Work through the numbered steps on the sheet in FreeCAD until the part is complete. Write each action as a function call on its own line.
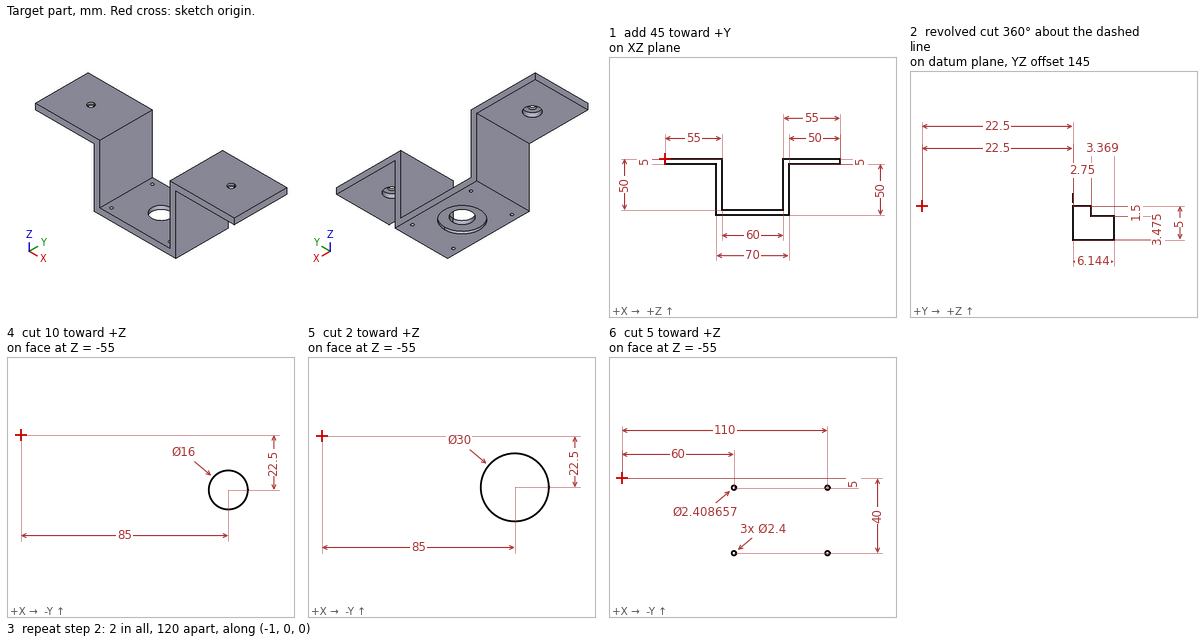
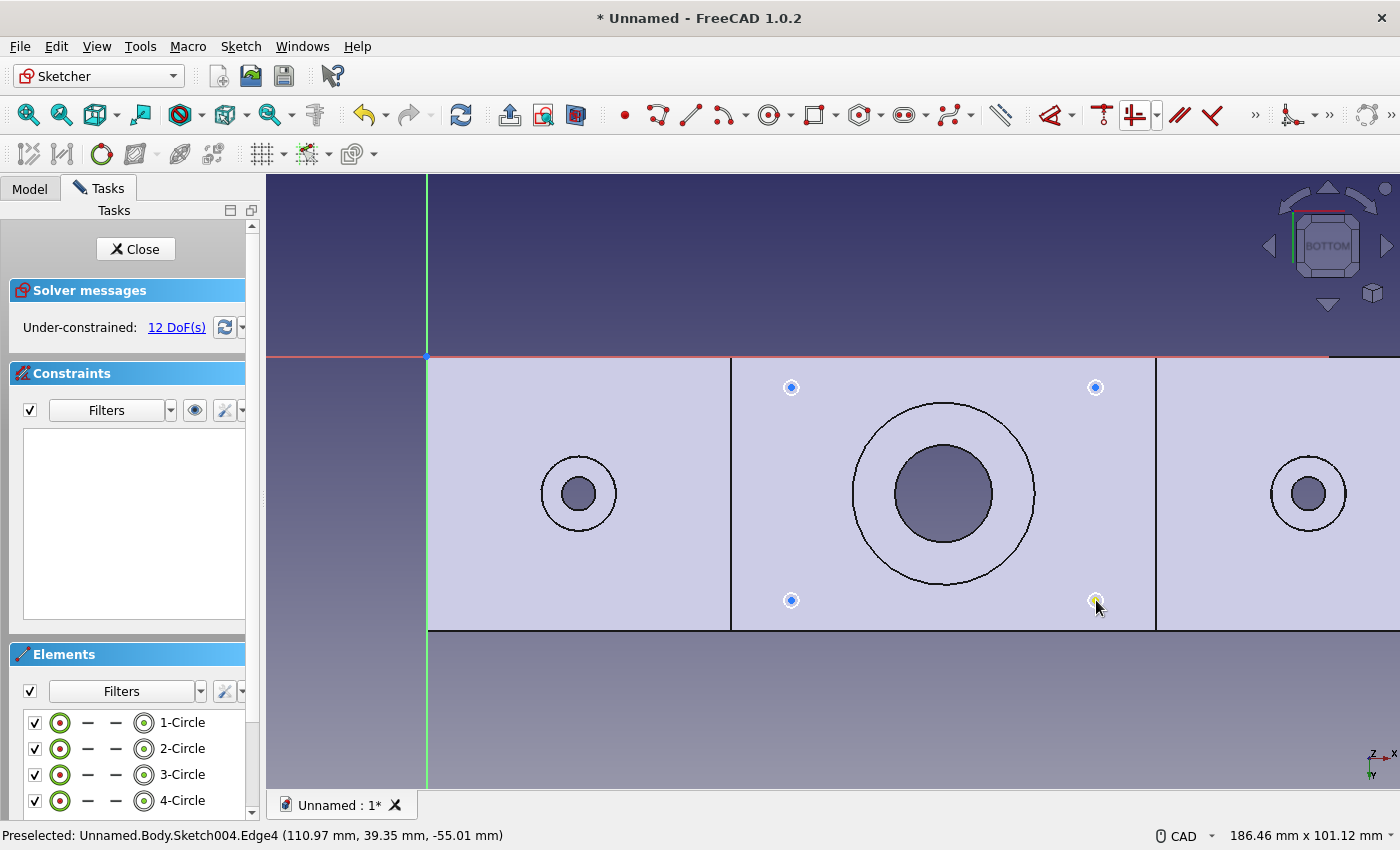
scroll(797, 595, up, 4)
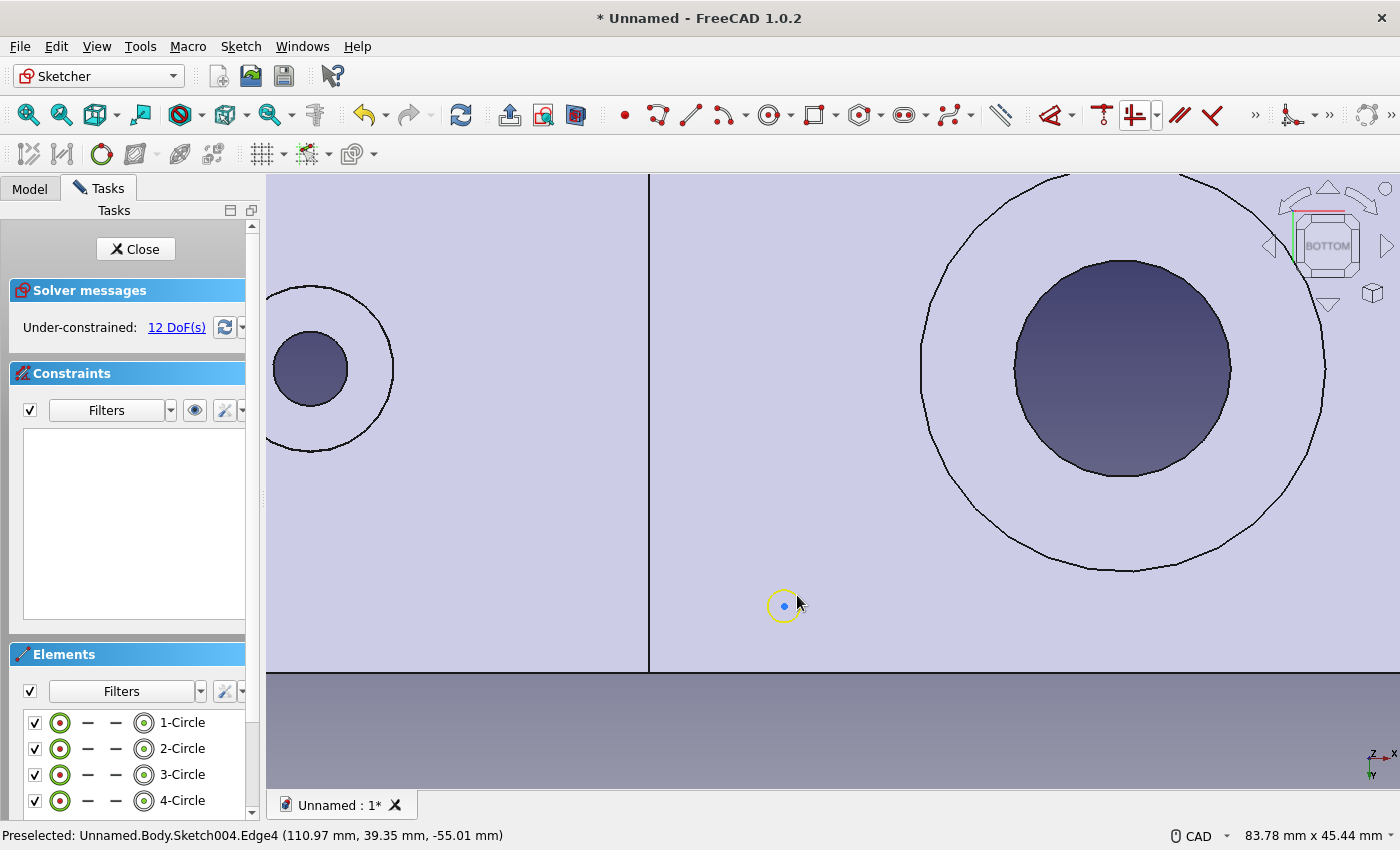
click(795, 595)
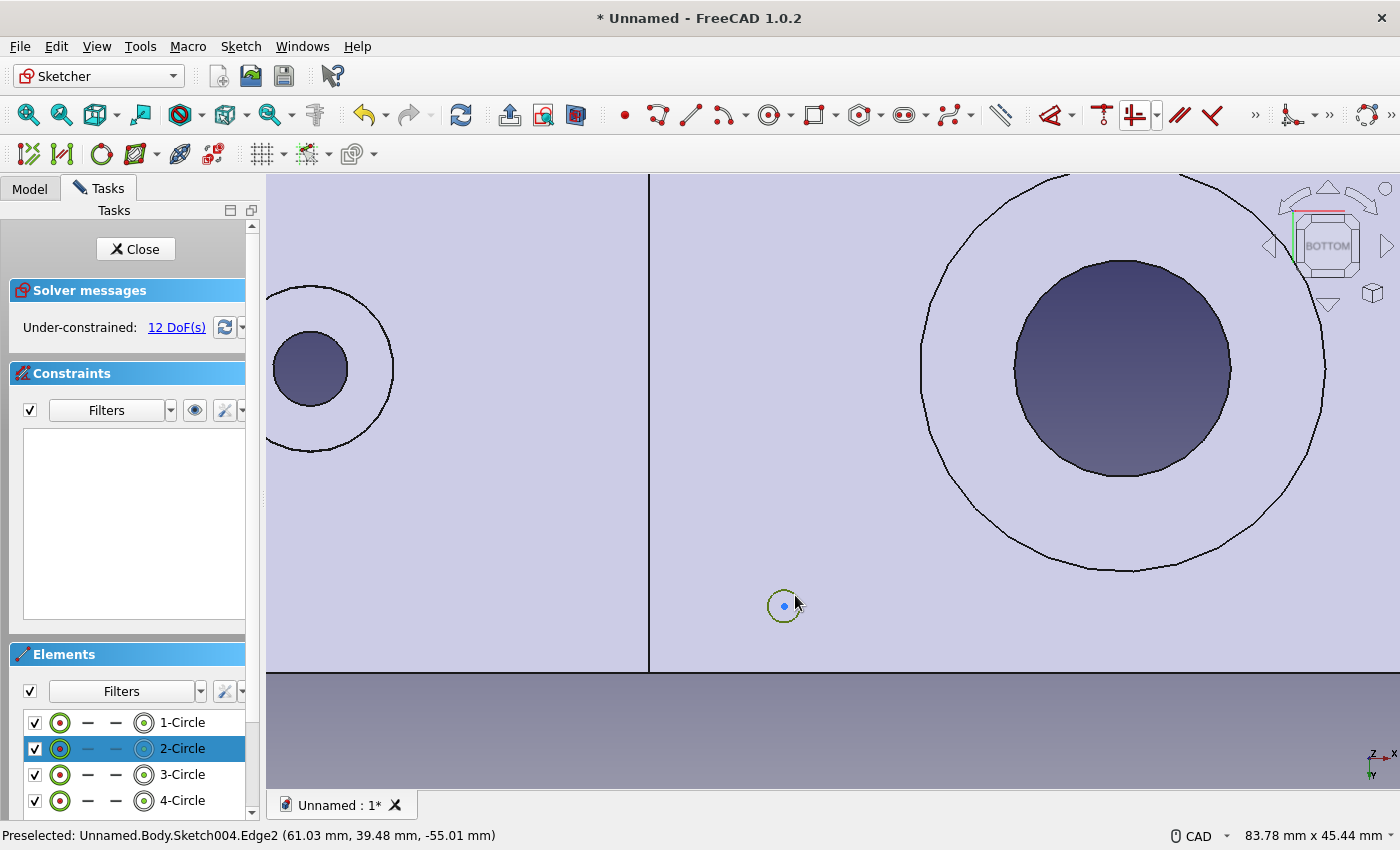
scroll(797, 594, down, 4)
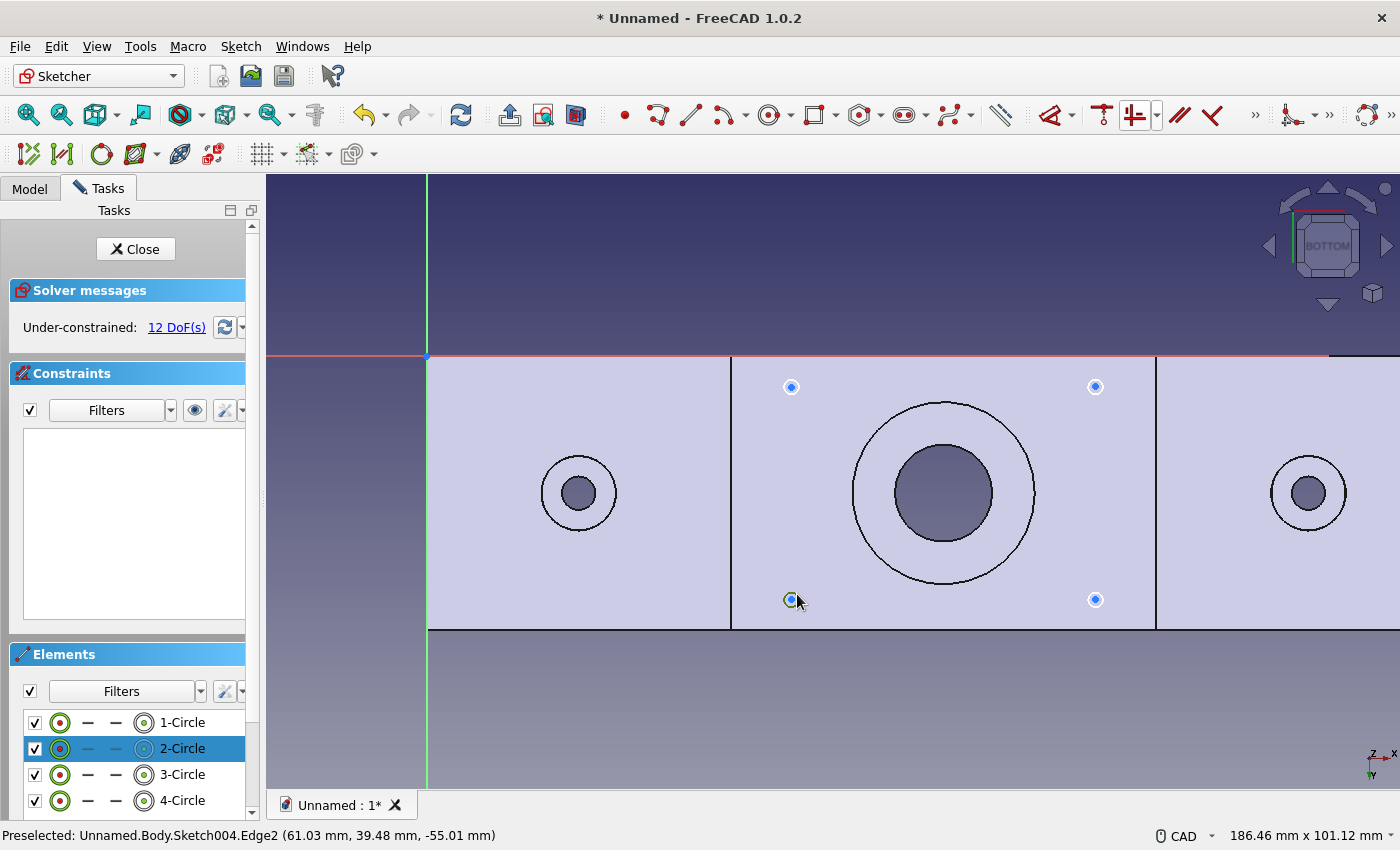
scroll(1101, 382, up, 4)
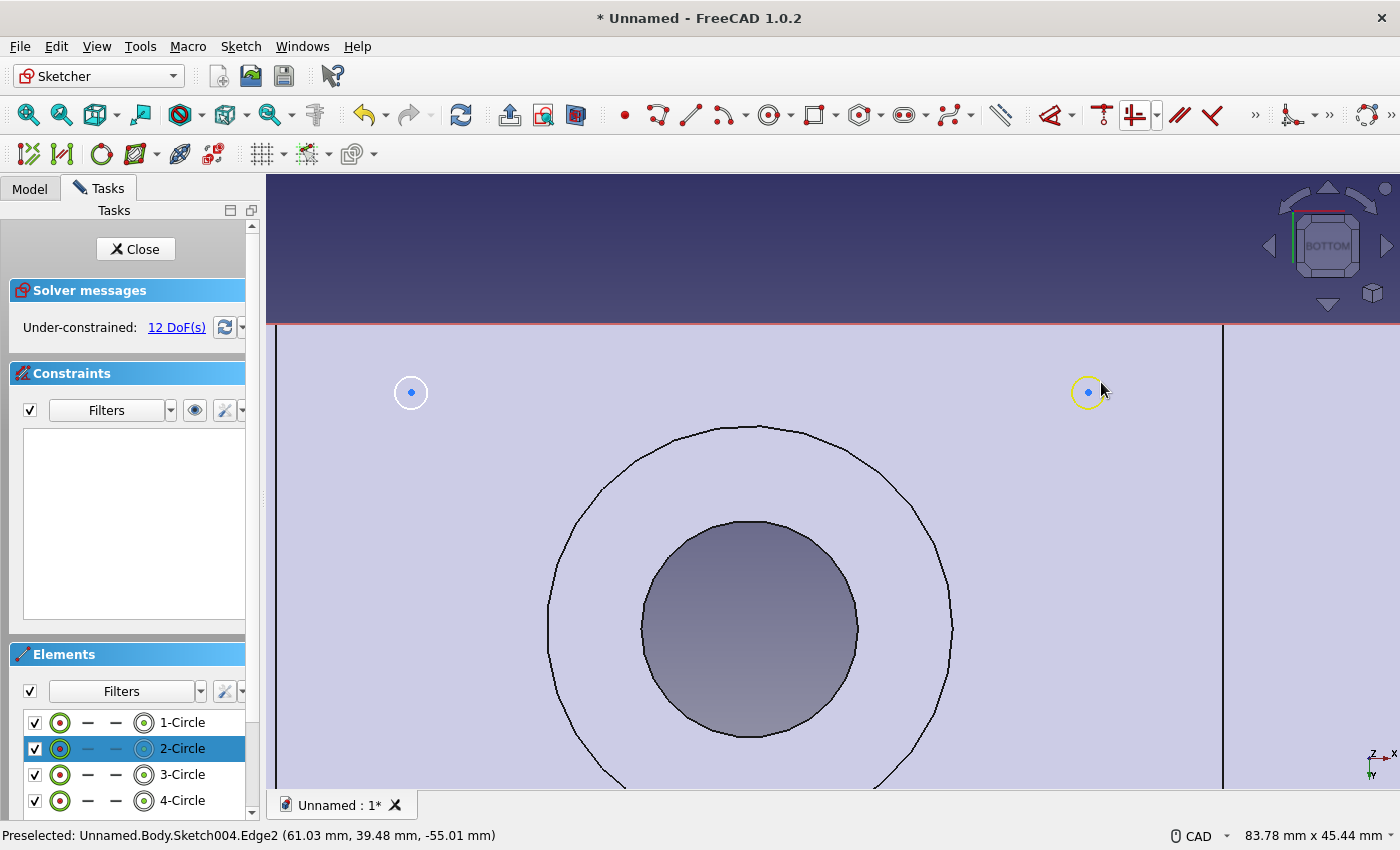
click(1099, 381)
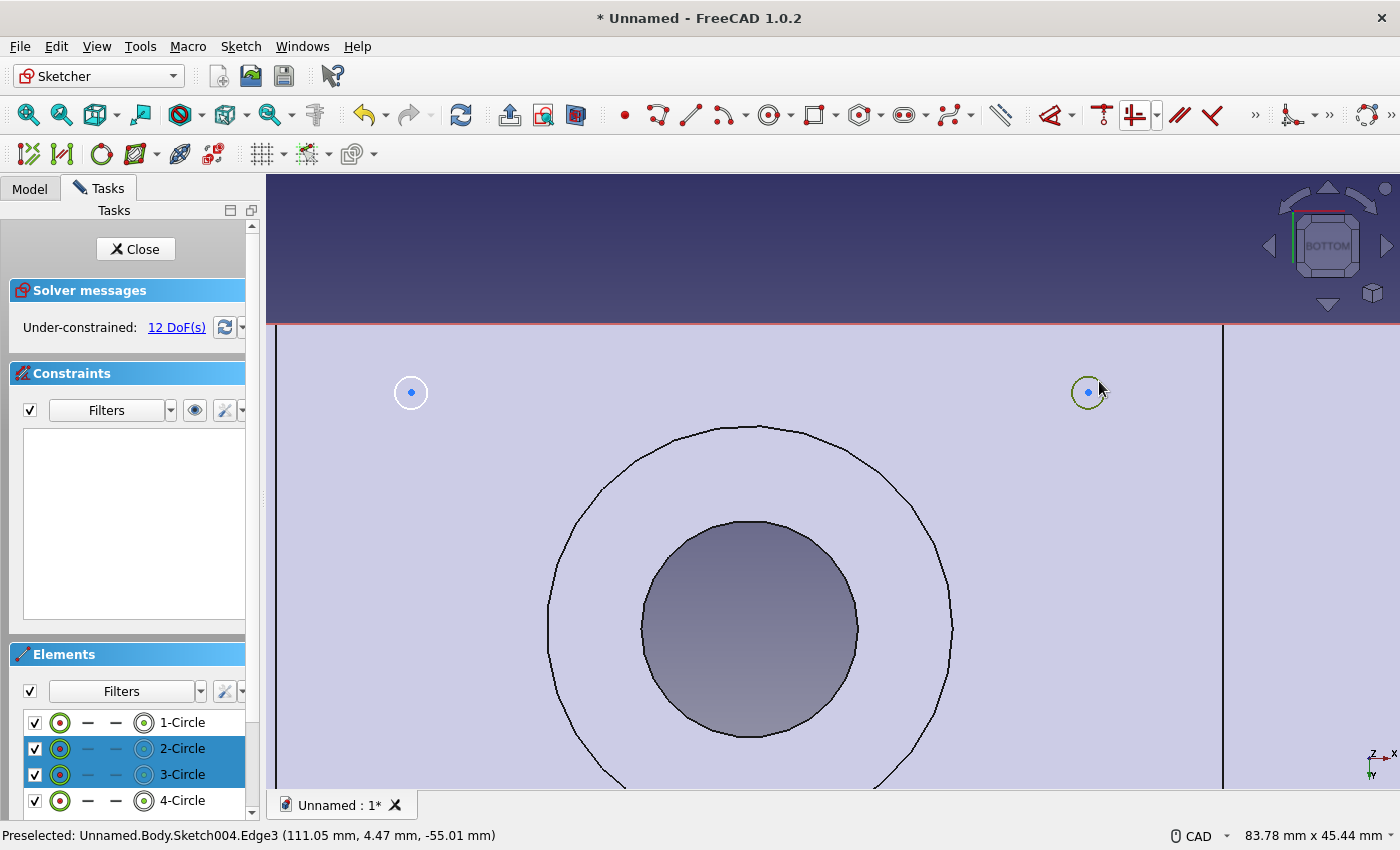
scroll(1101, 382, down, 4)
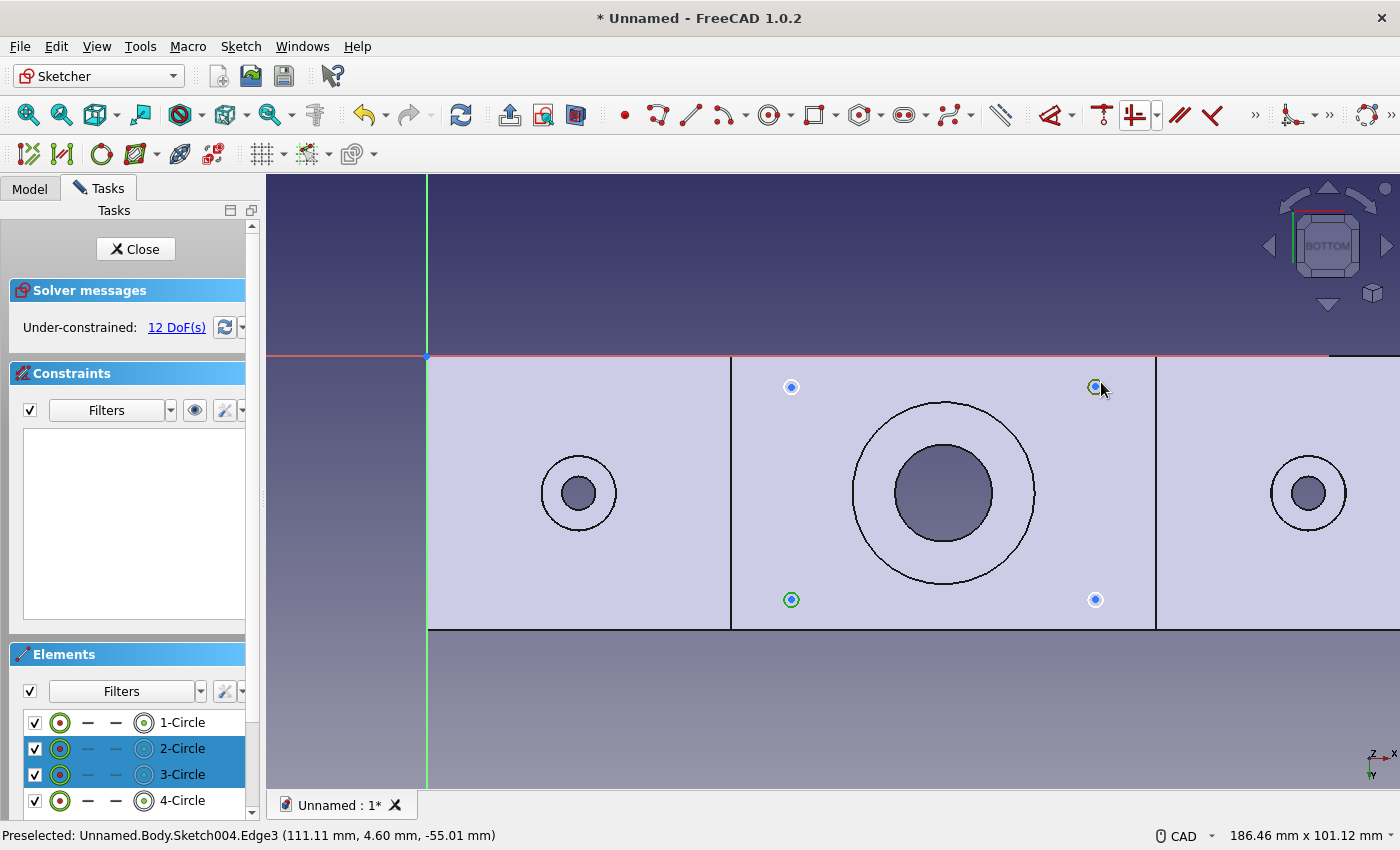
scroll(1101, 595, up, 4)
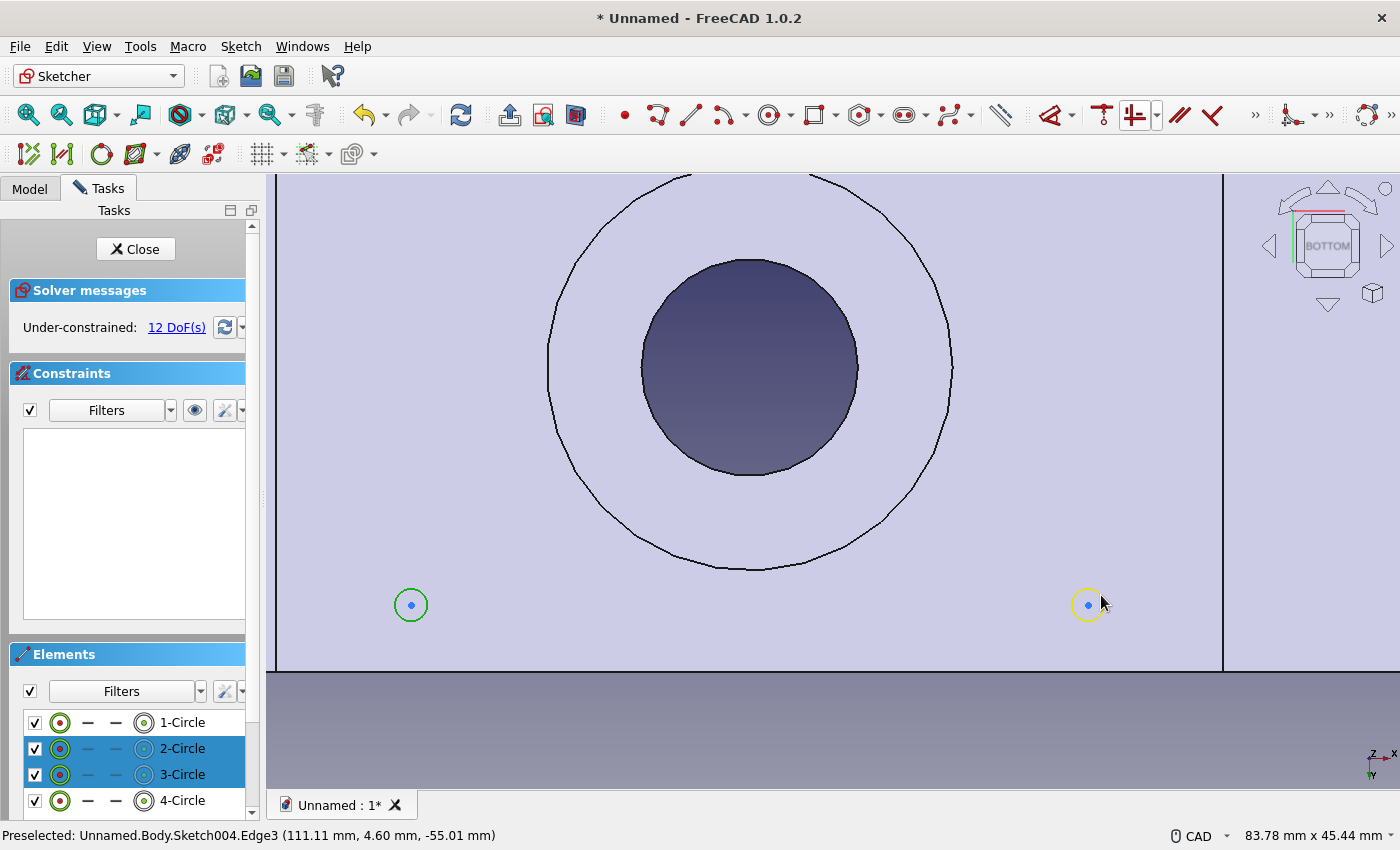
click(1099, 594)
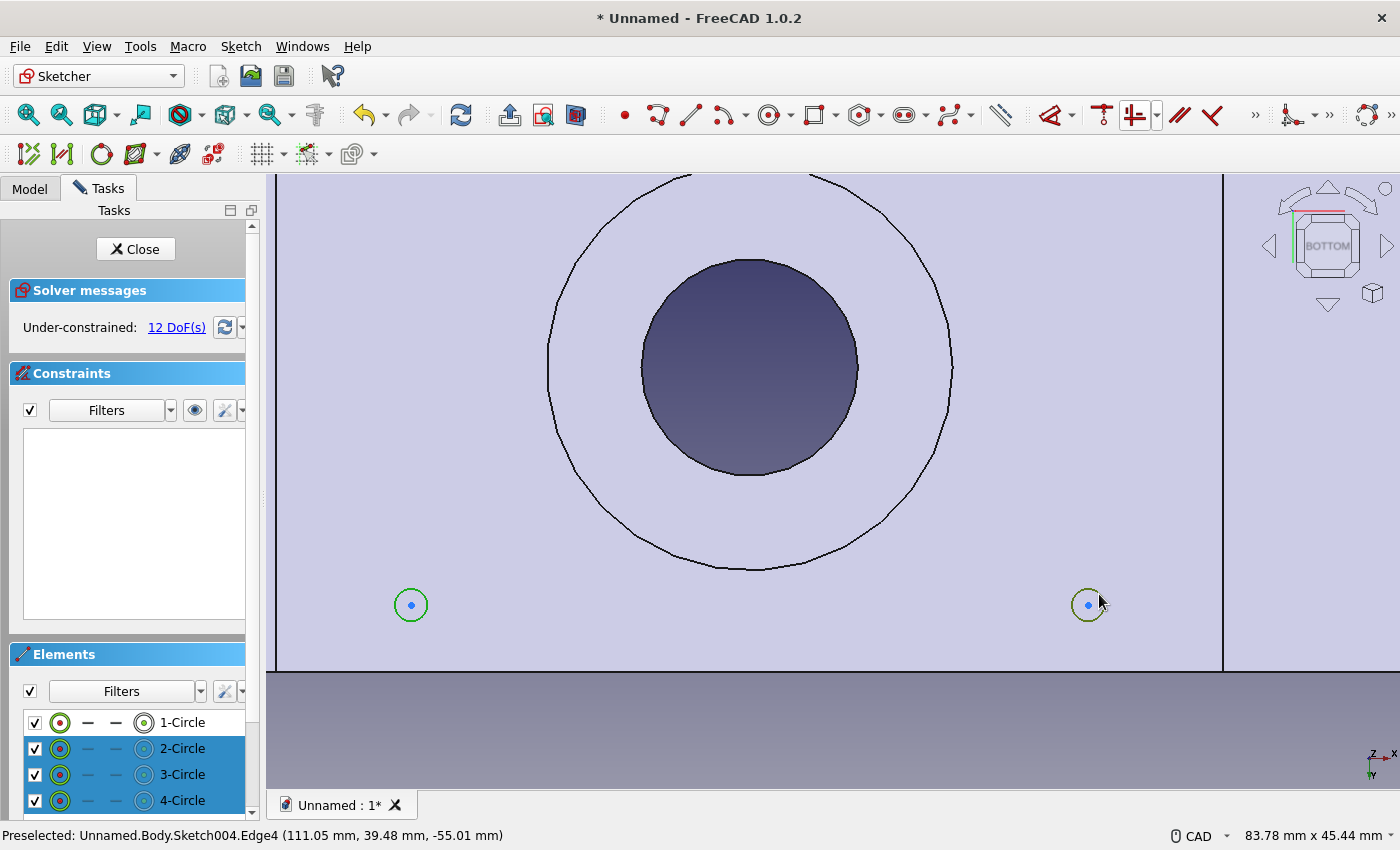
key(e)